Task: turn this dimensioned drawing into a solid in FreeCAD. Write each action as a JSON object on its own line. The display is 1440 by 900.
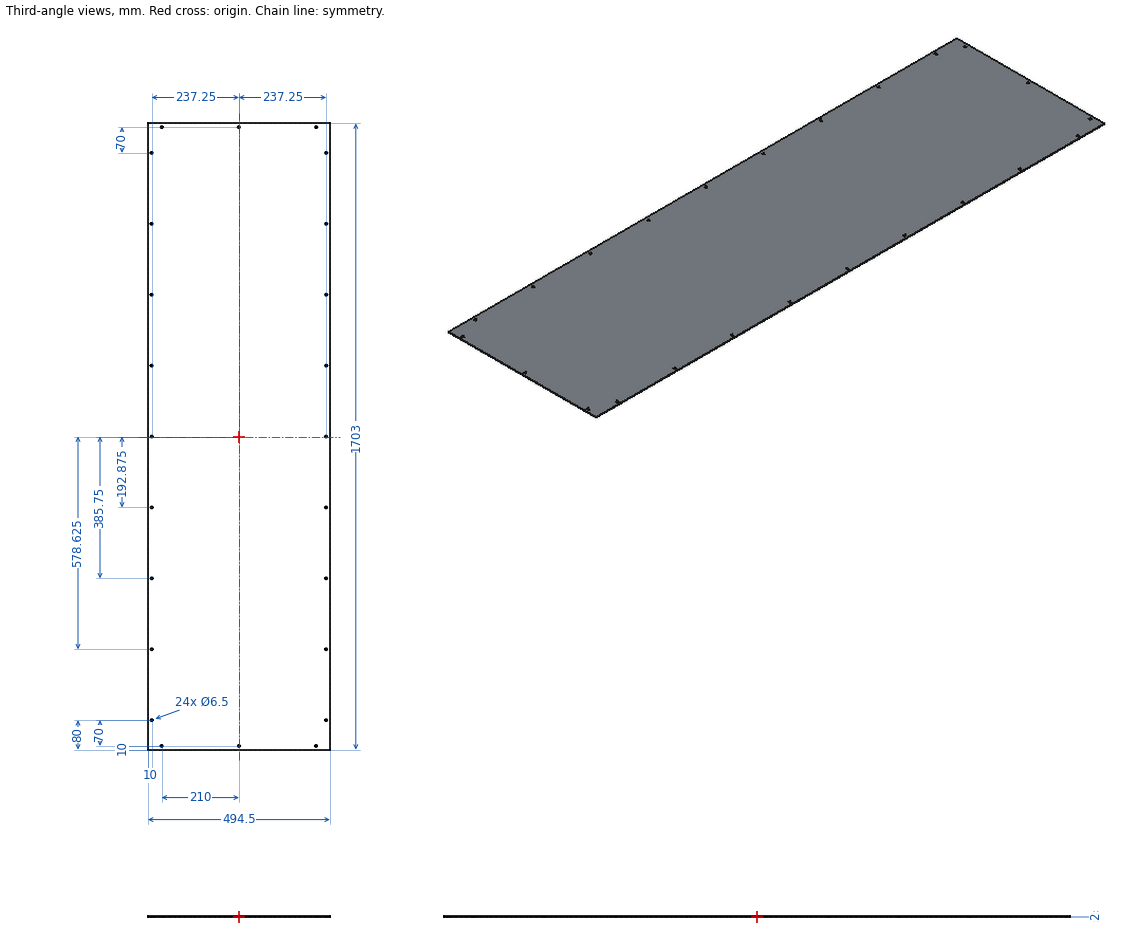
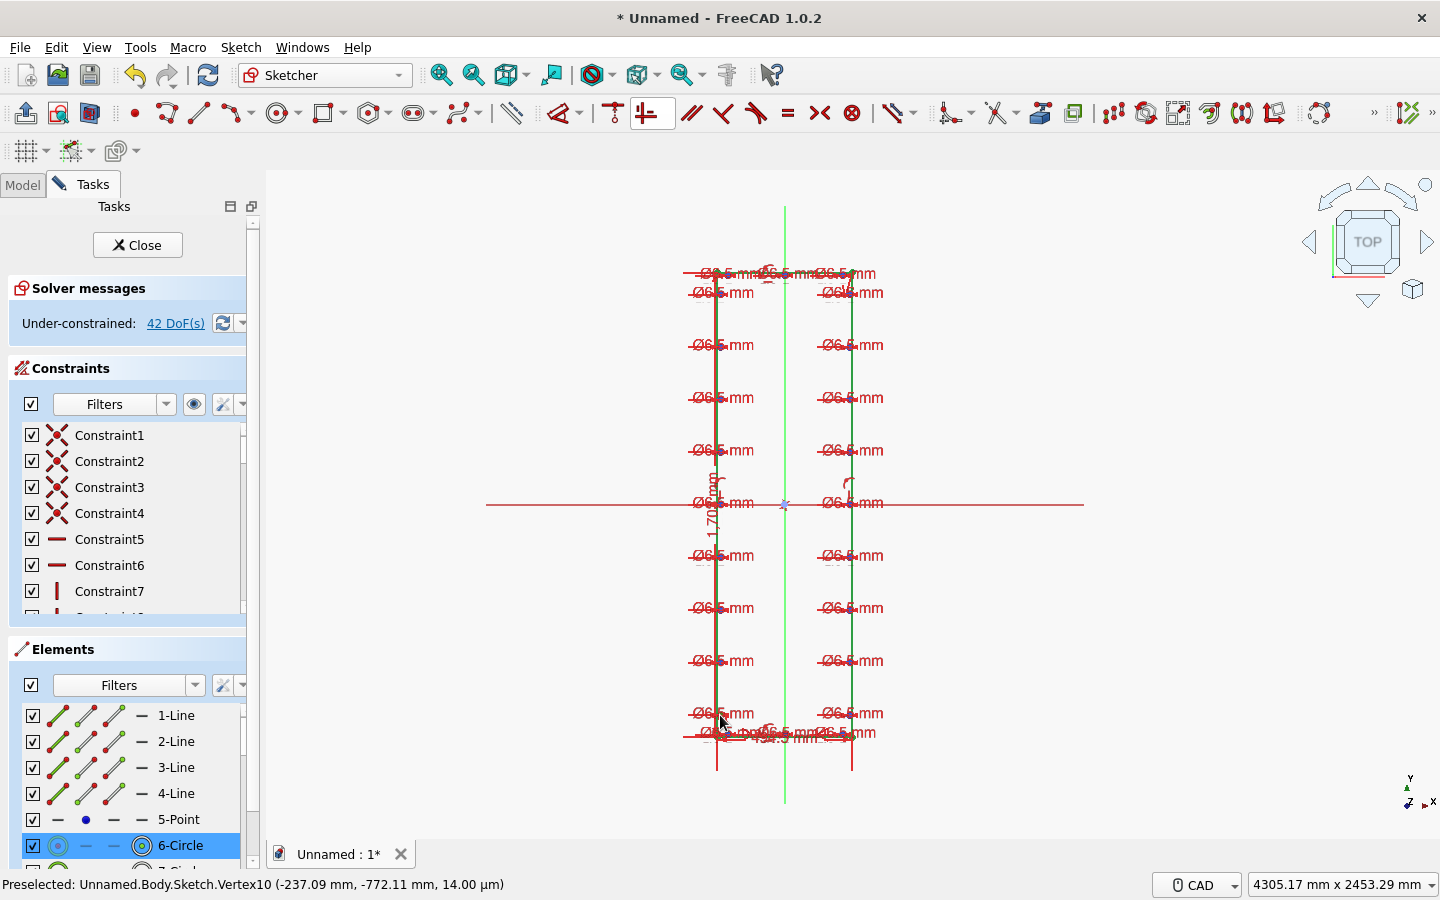
{"action": "left_click", "coordinate": [850, 715]}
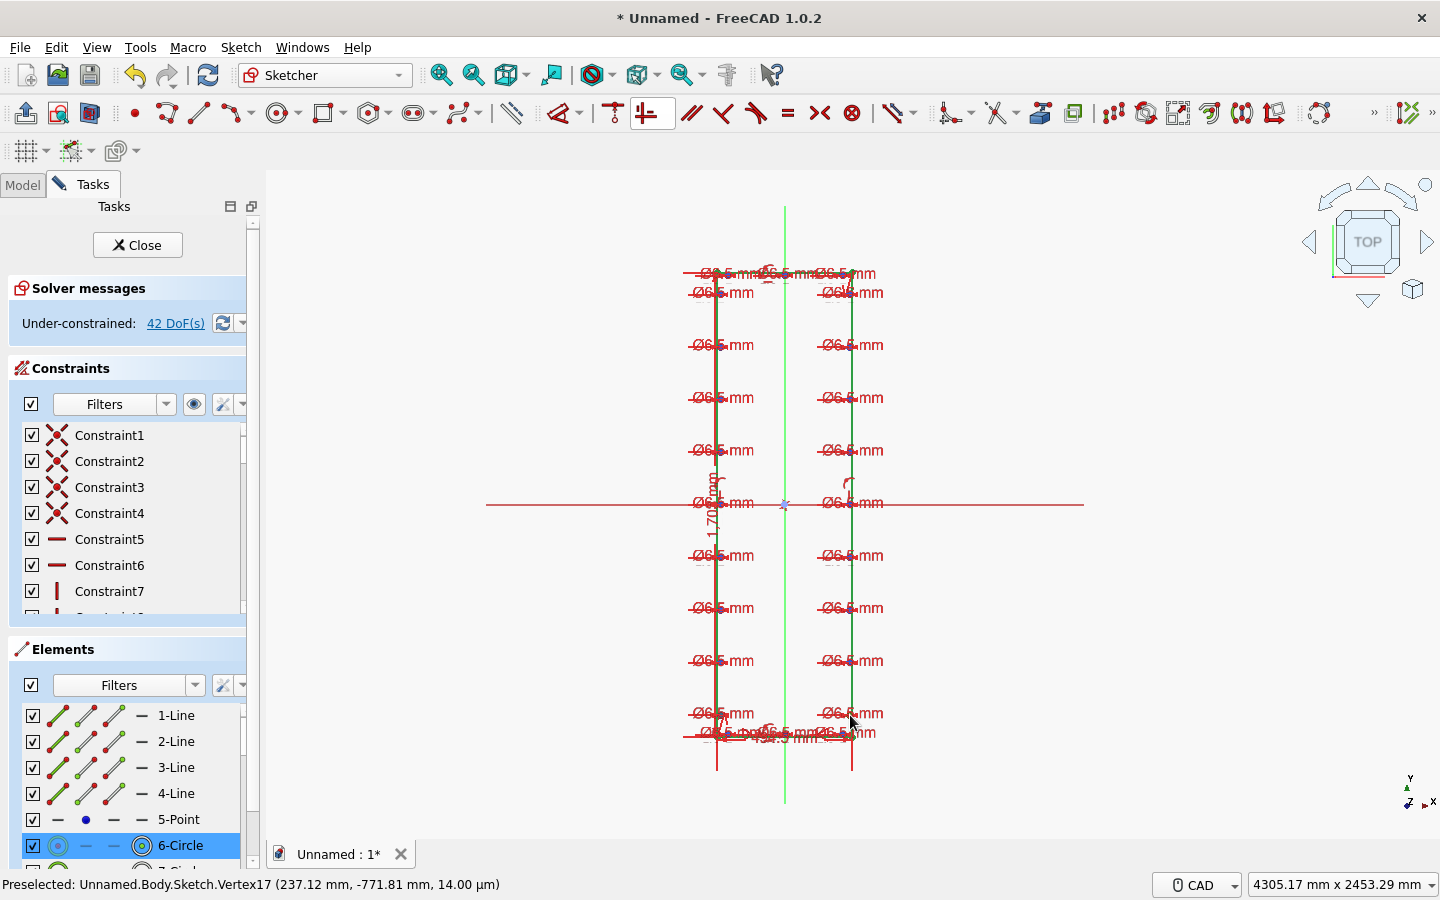
{"action": "left_click", "coordinate": [785, 767]}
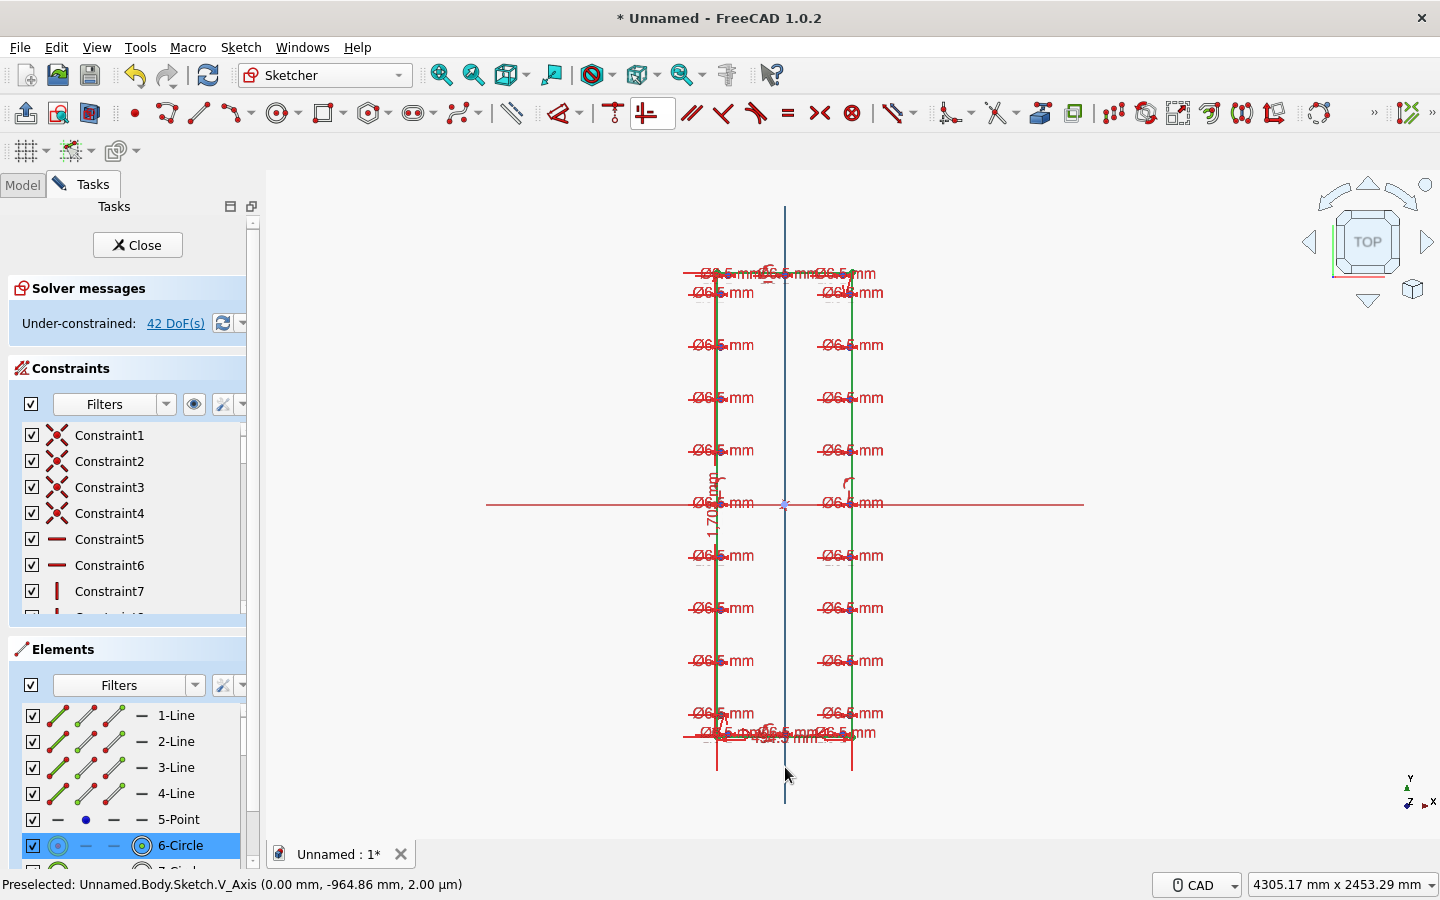
{"action": "left_click", "coordinate": [820, 114]}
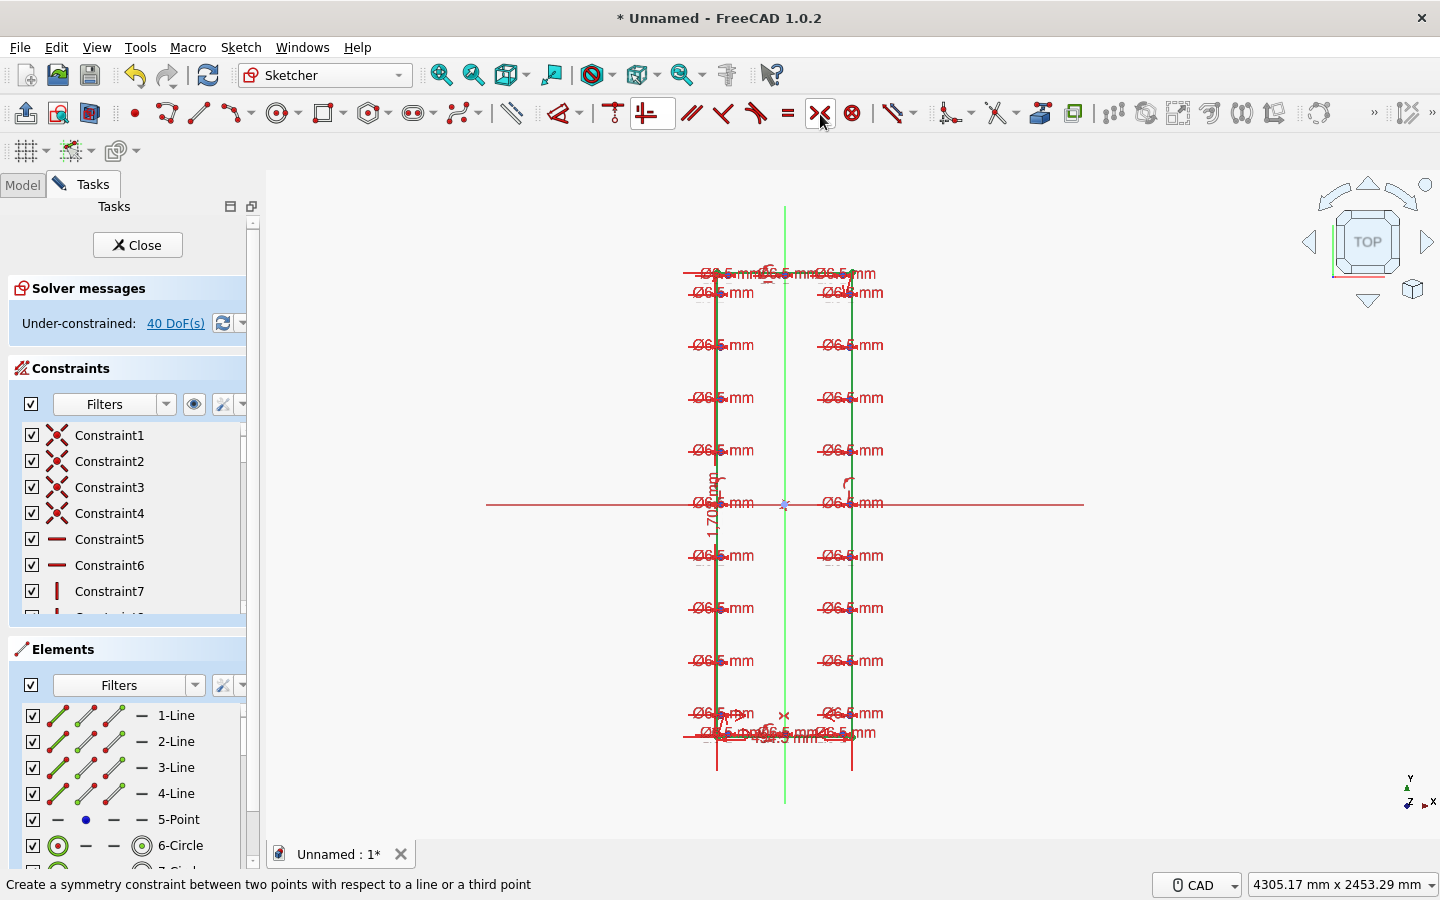
{"action": "left_click", "coordinate": [720, 663]}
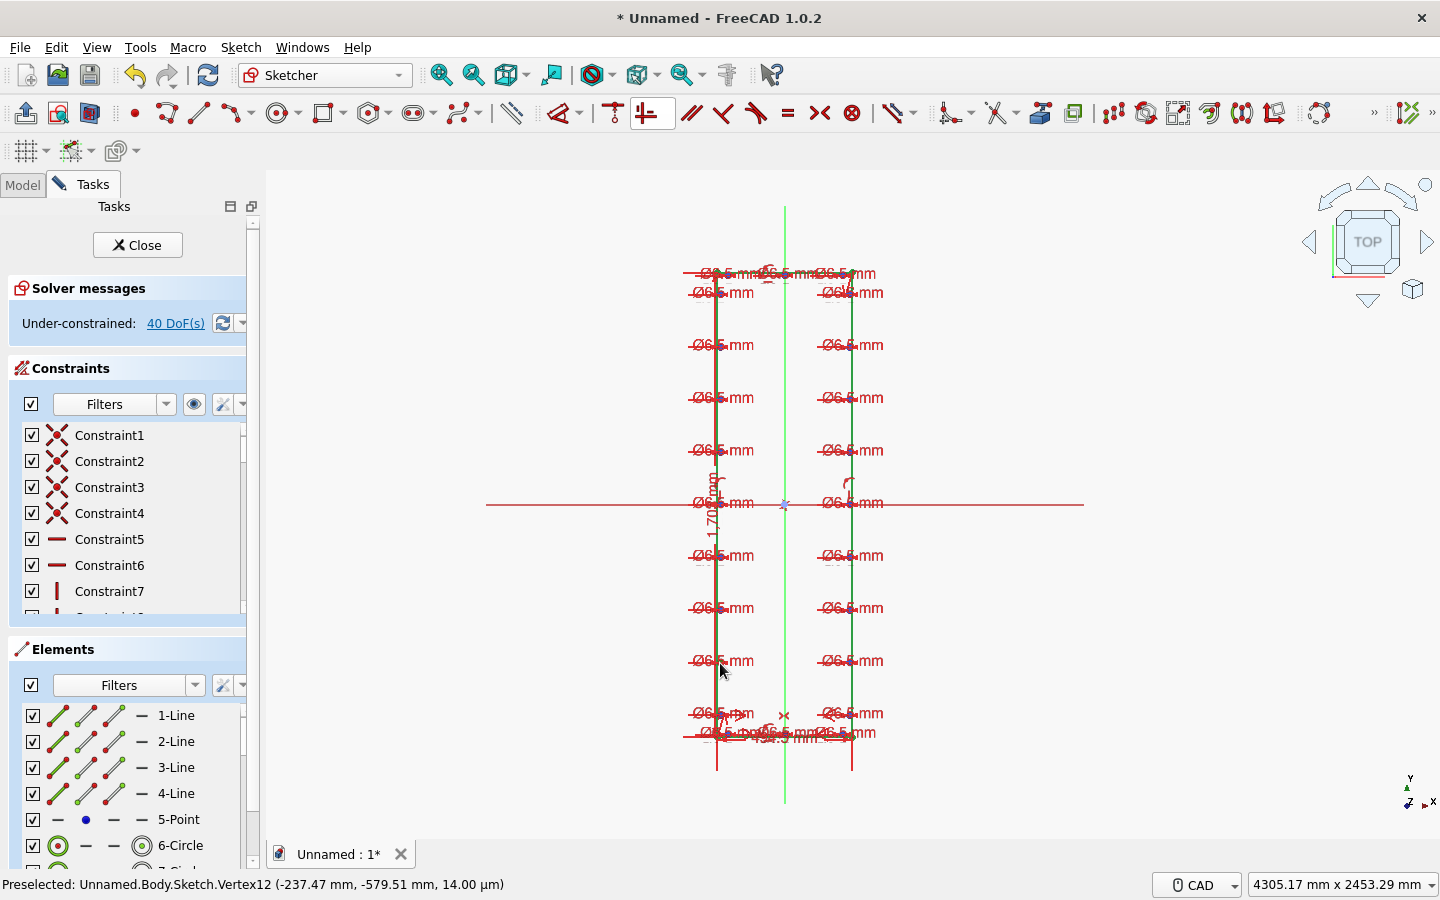
{"action": "left_click", "coordinate": [850, 663]}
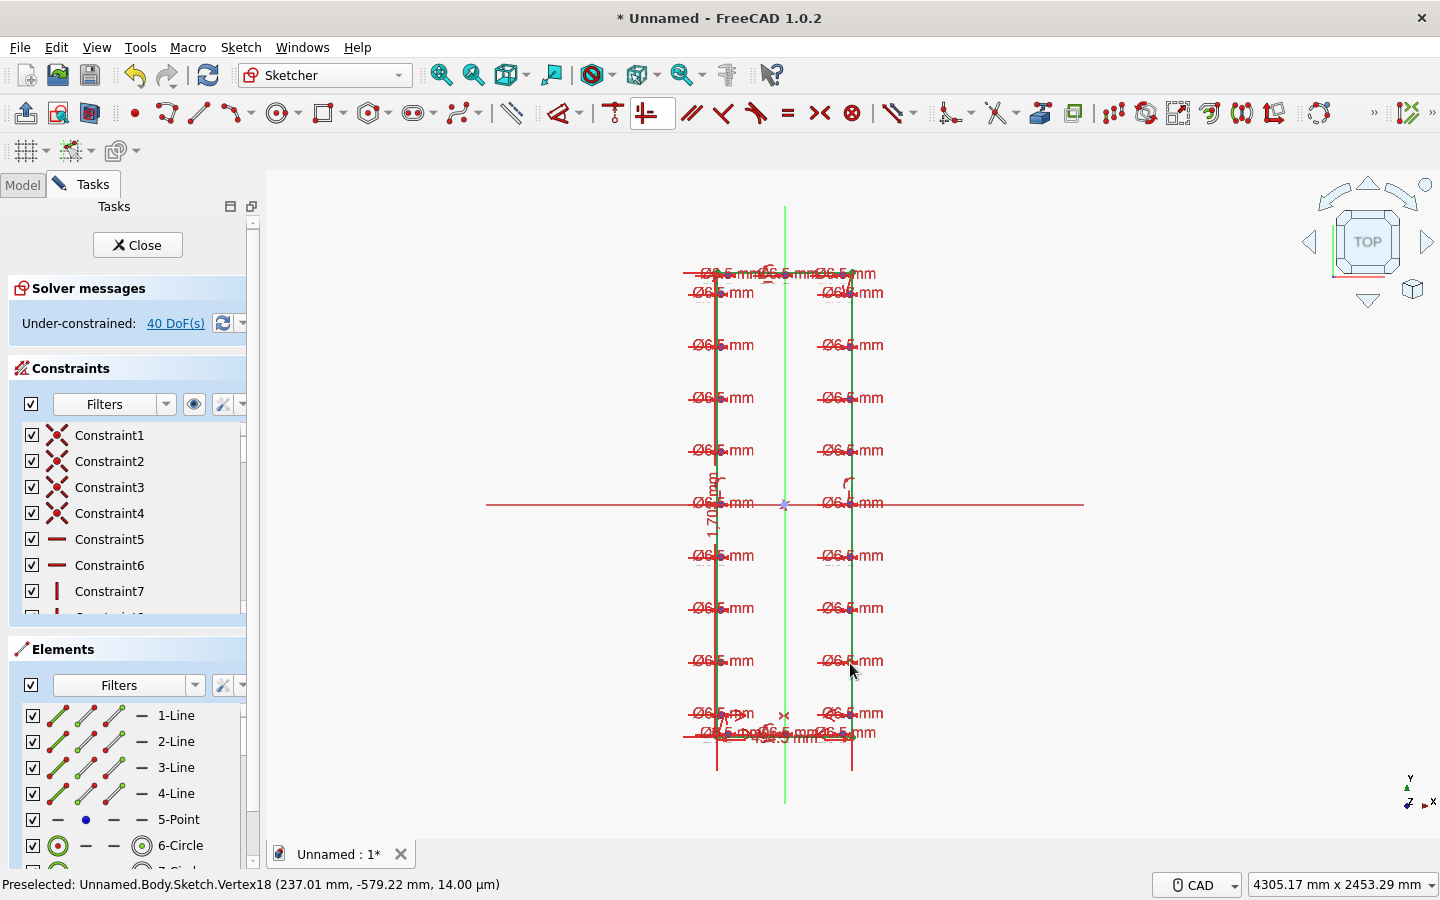
{"action": "left_click", "coordinate": [785, 767]}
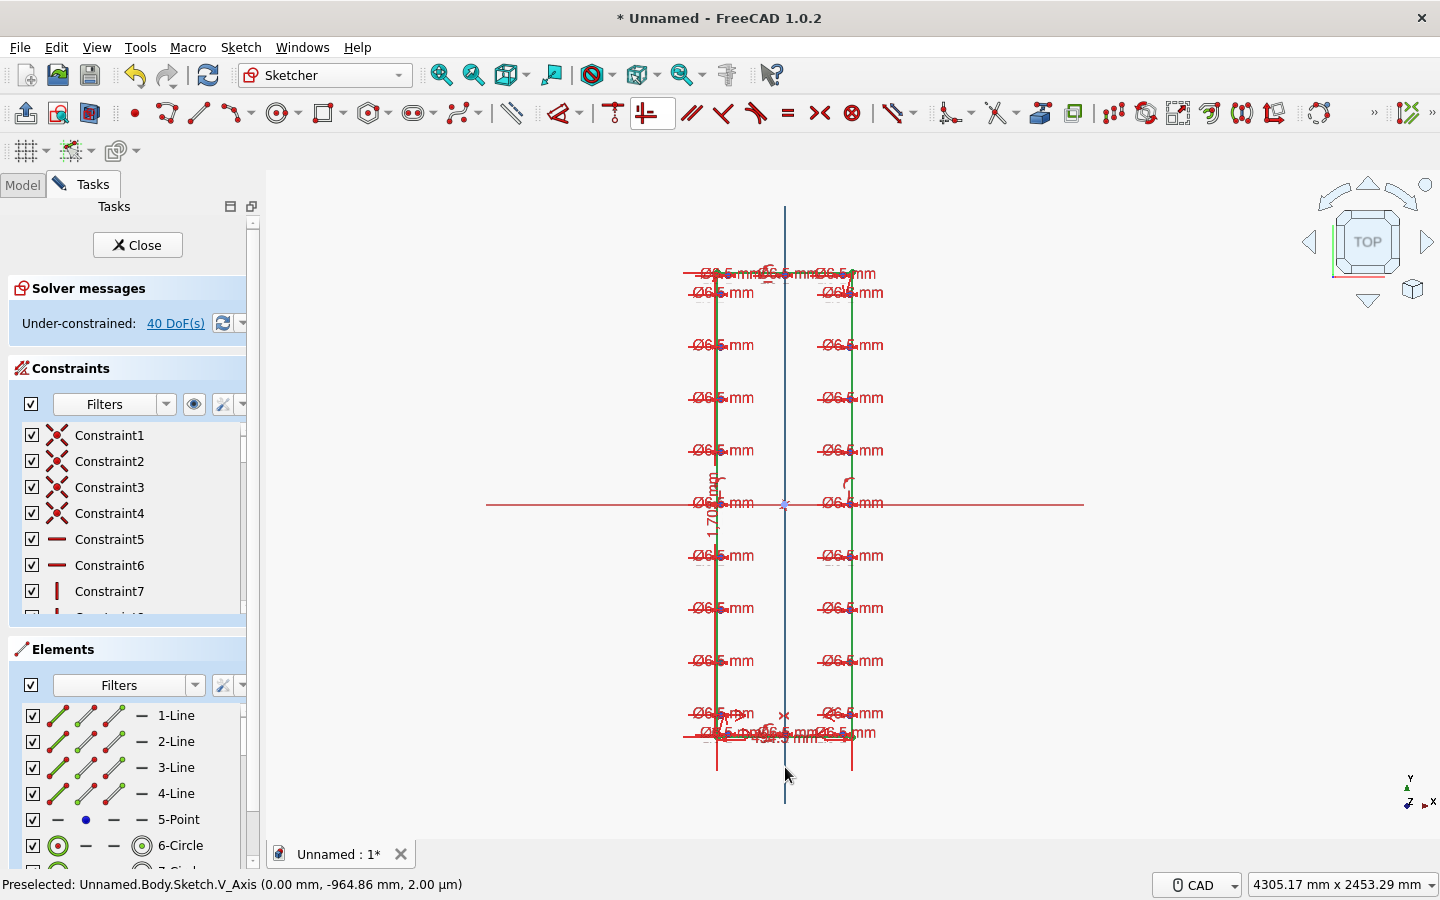
{"action": "left_click", "coordinate": [820, 114]}